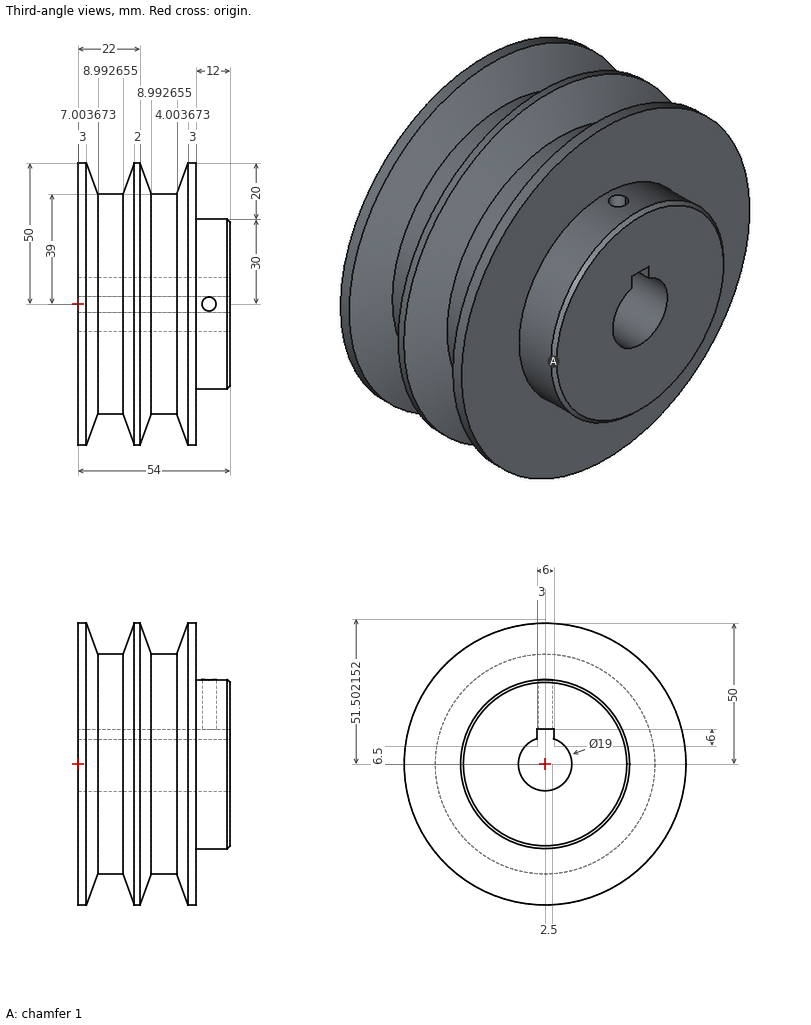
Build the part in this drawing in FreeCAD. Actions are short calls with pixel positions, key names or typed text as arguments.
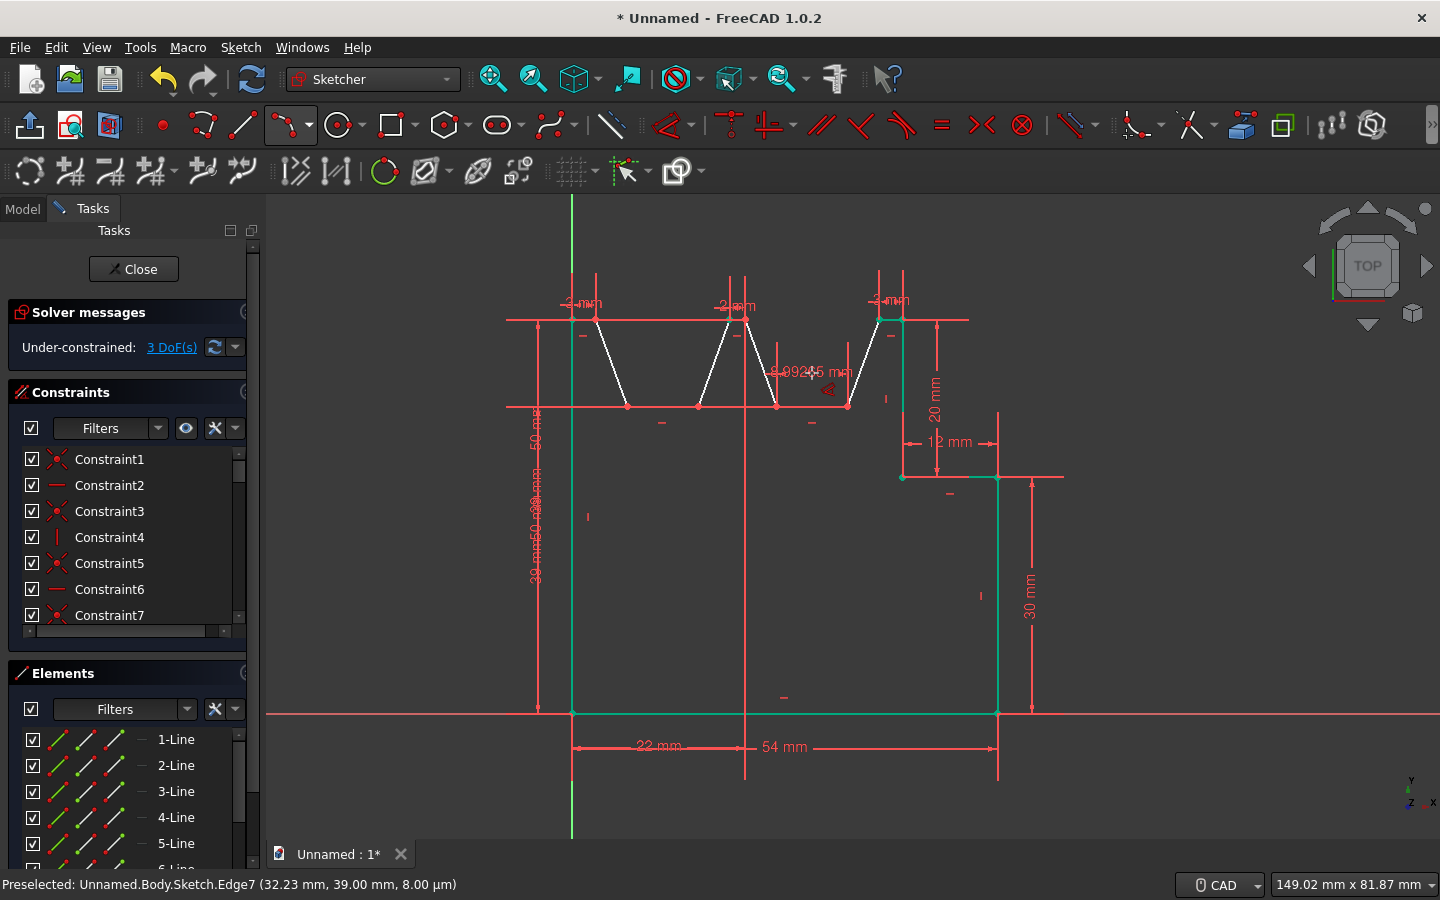
click(677, 407)
click(663, 373)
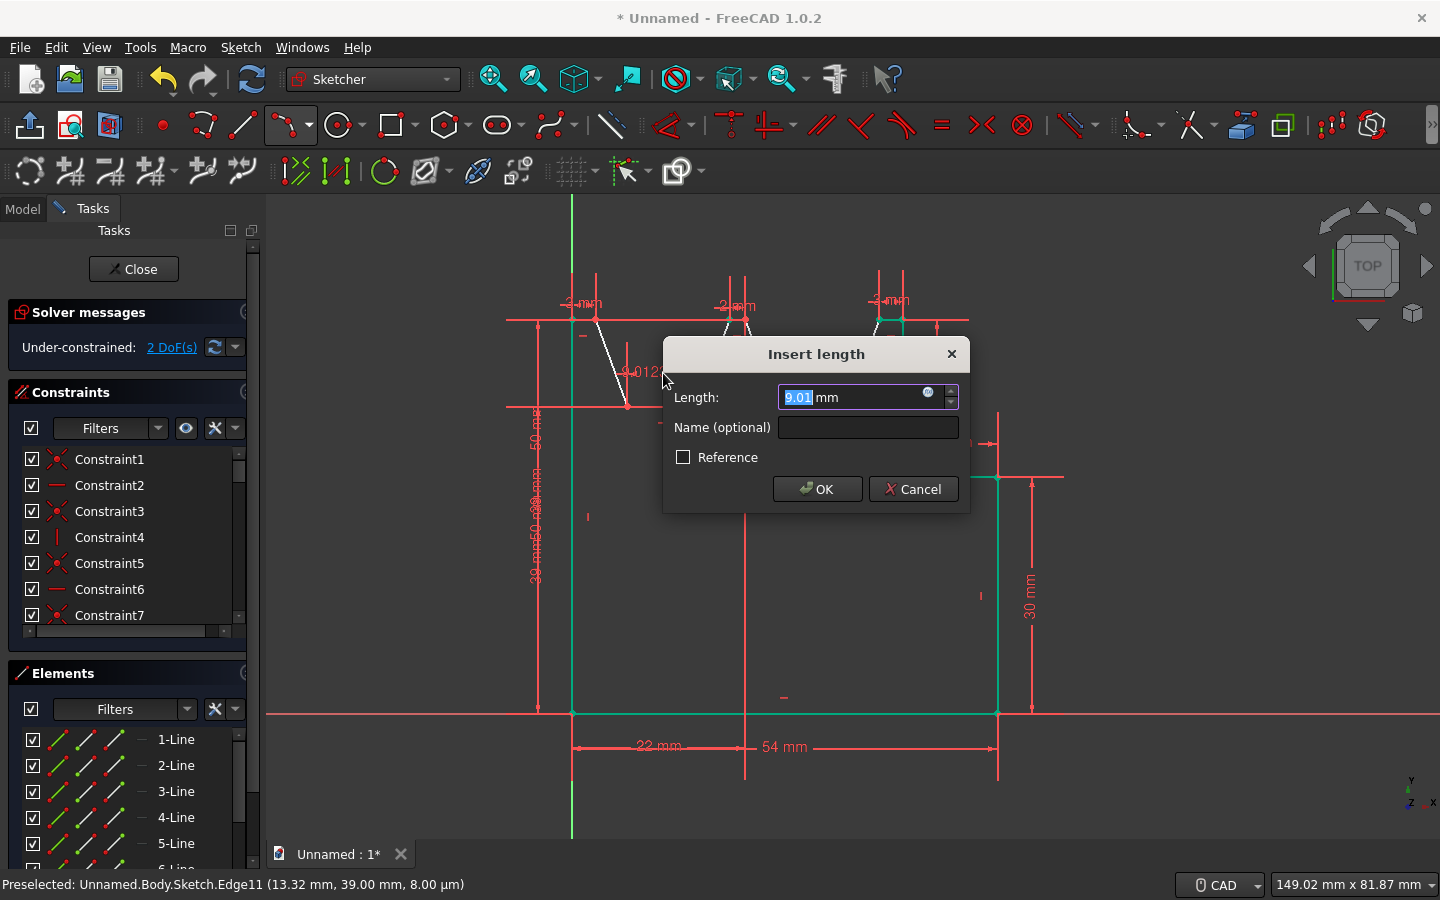
text(8.992655)
key(Return)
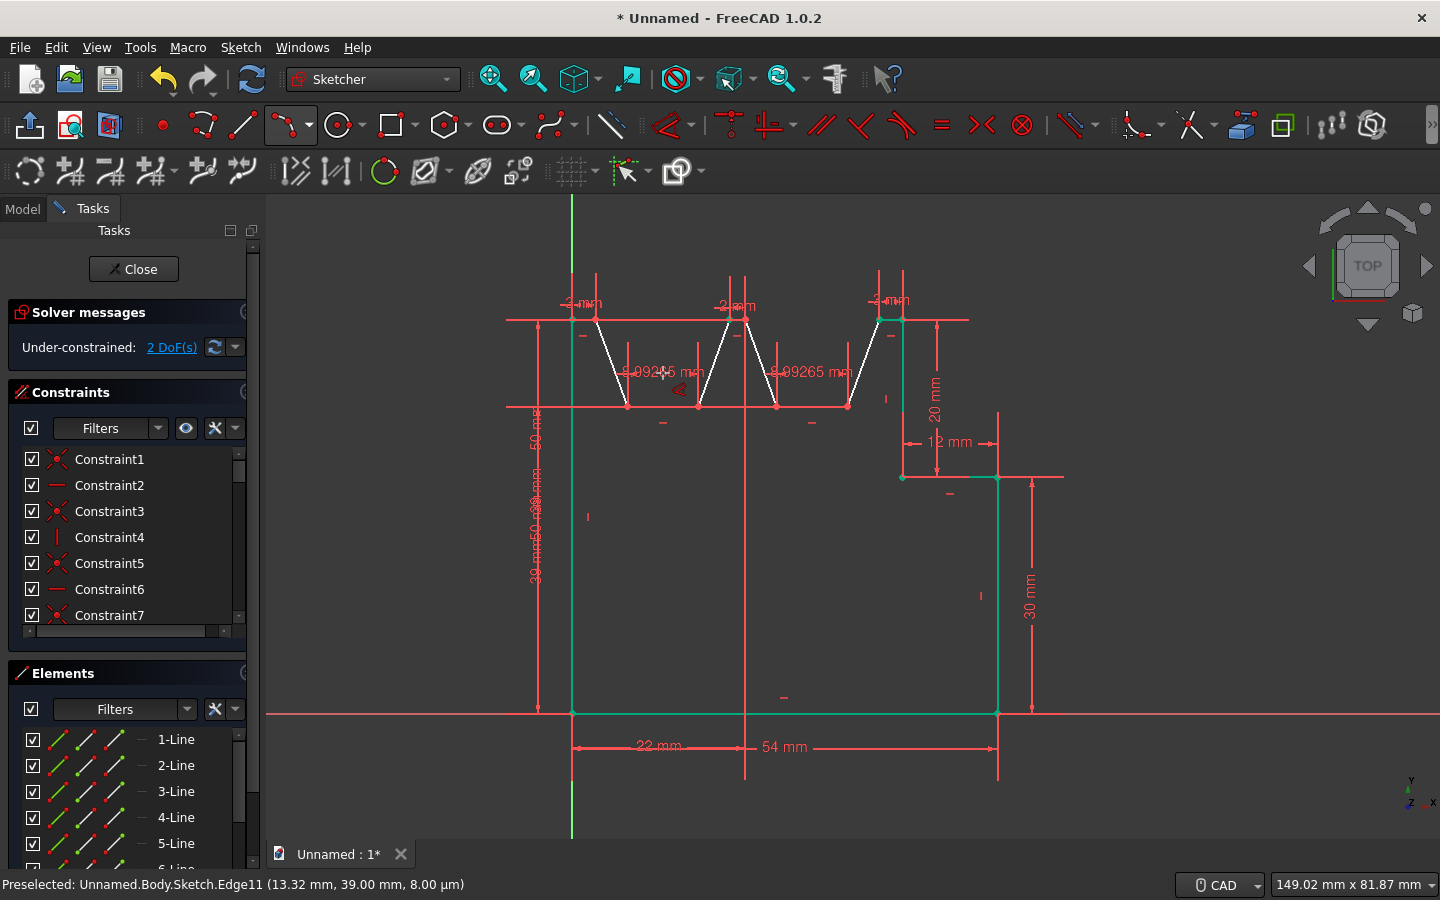
click(628, 407)
click(587, 748)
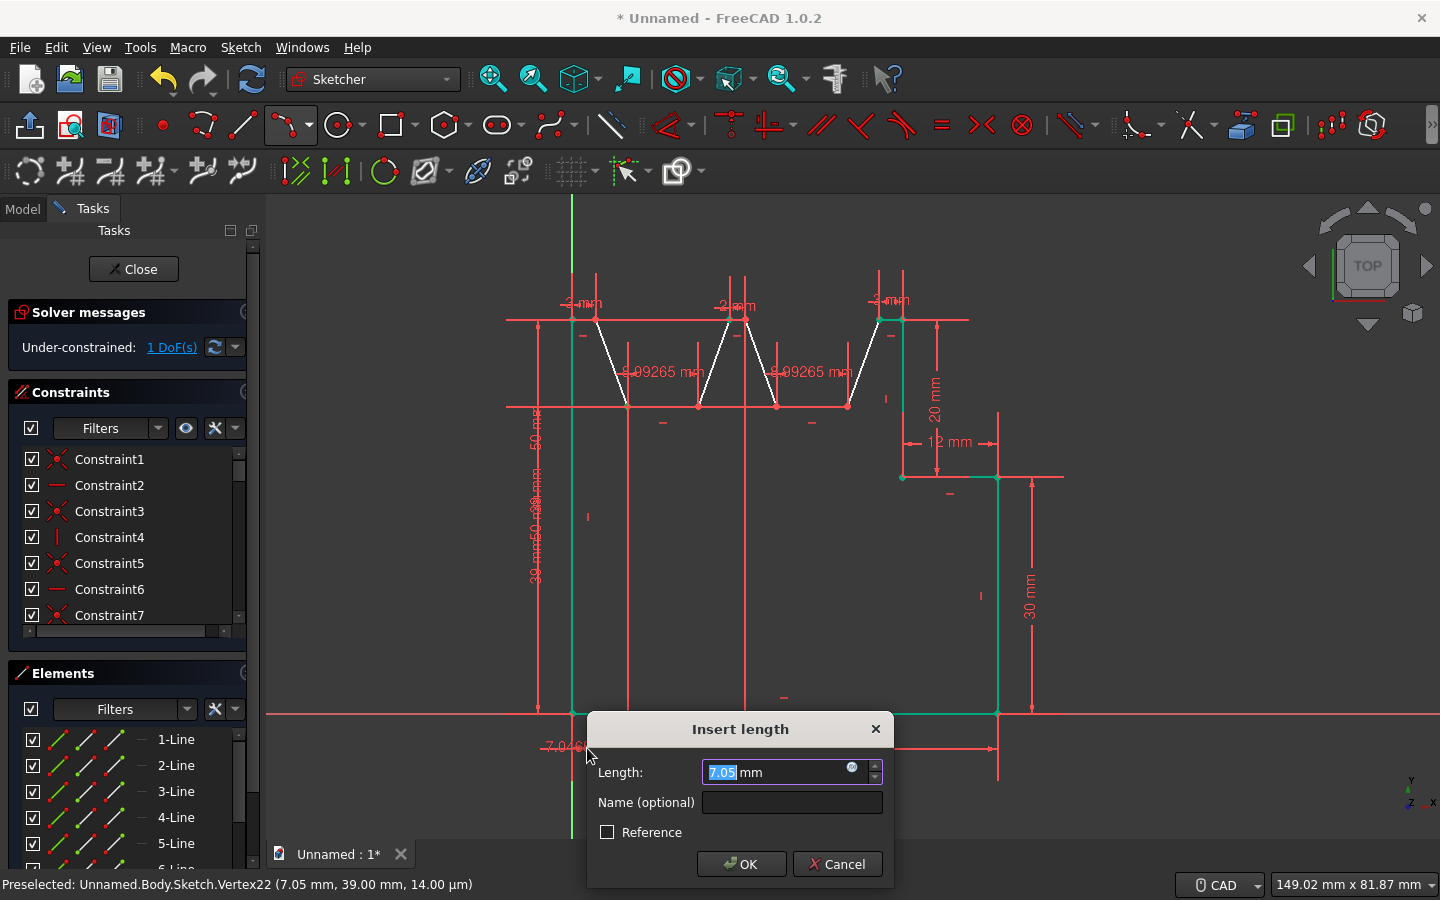
text(7.003673)
key(Return)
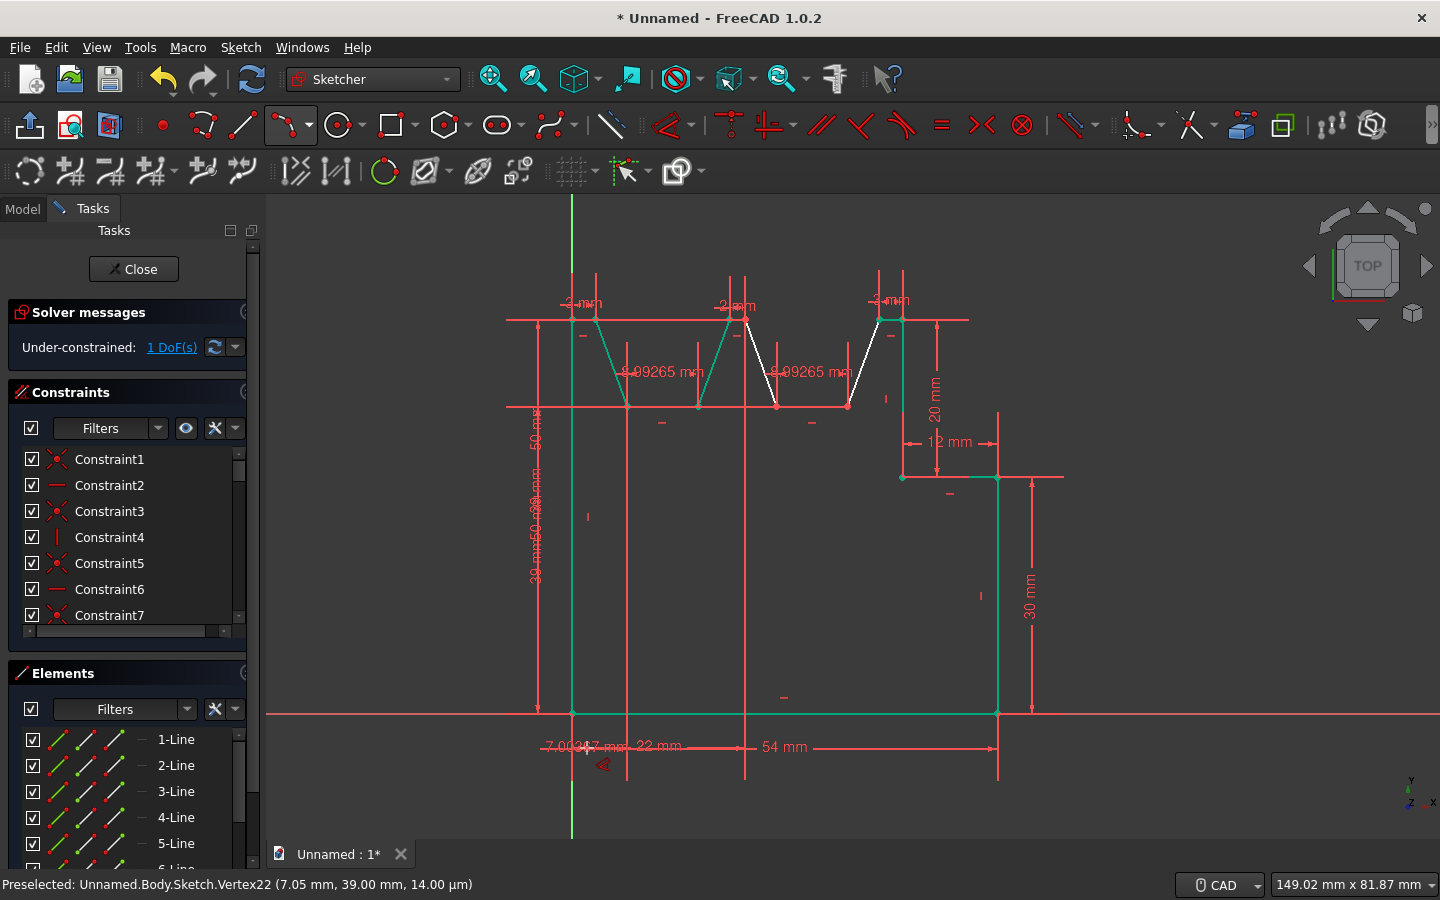
scroll(870, 346, up, 2)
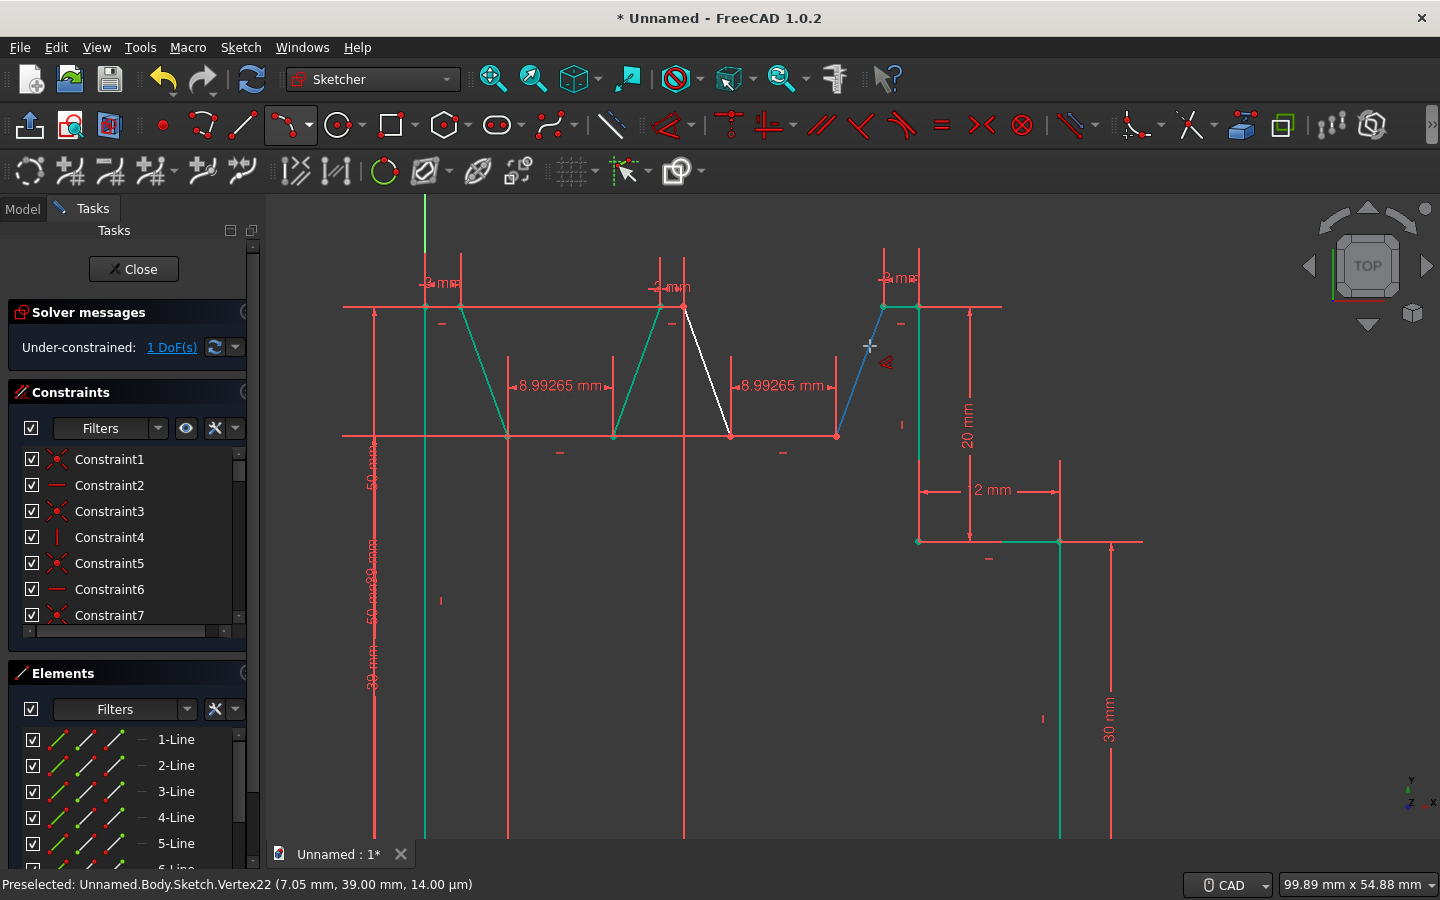
click(869, 346)
click(860, 470)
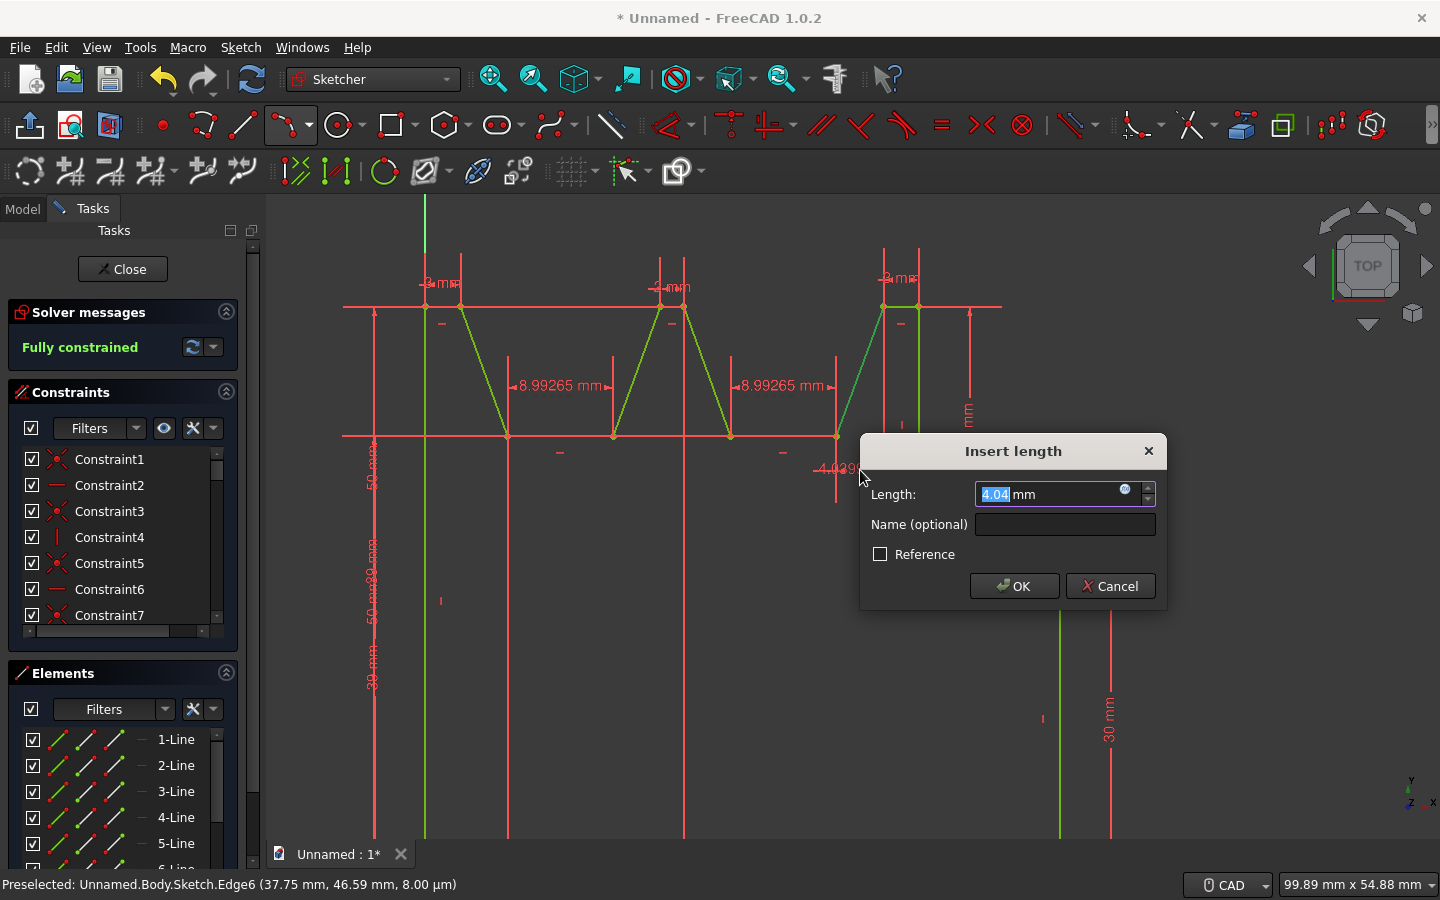
text(4.003673)
key(Return)
key(Escape)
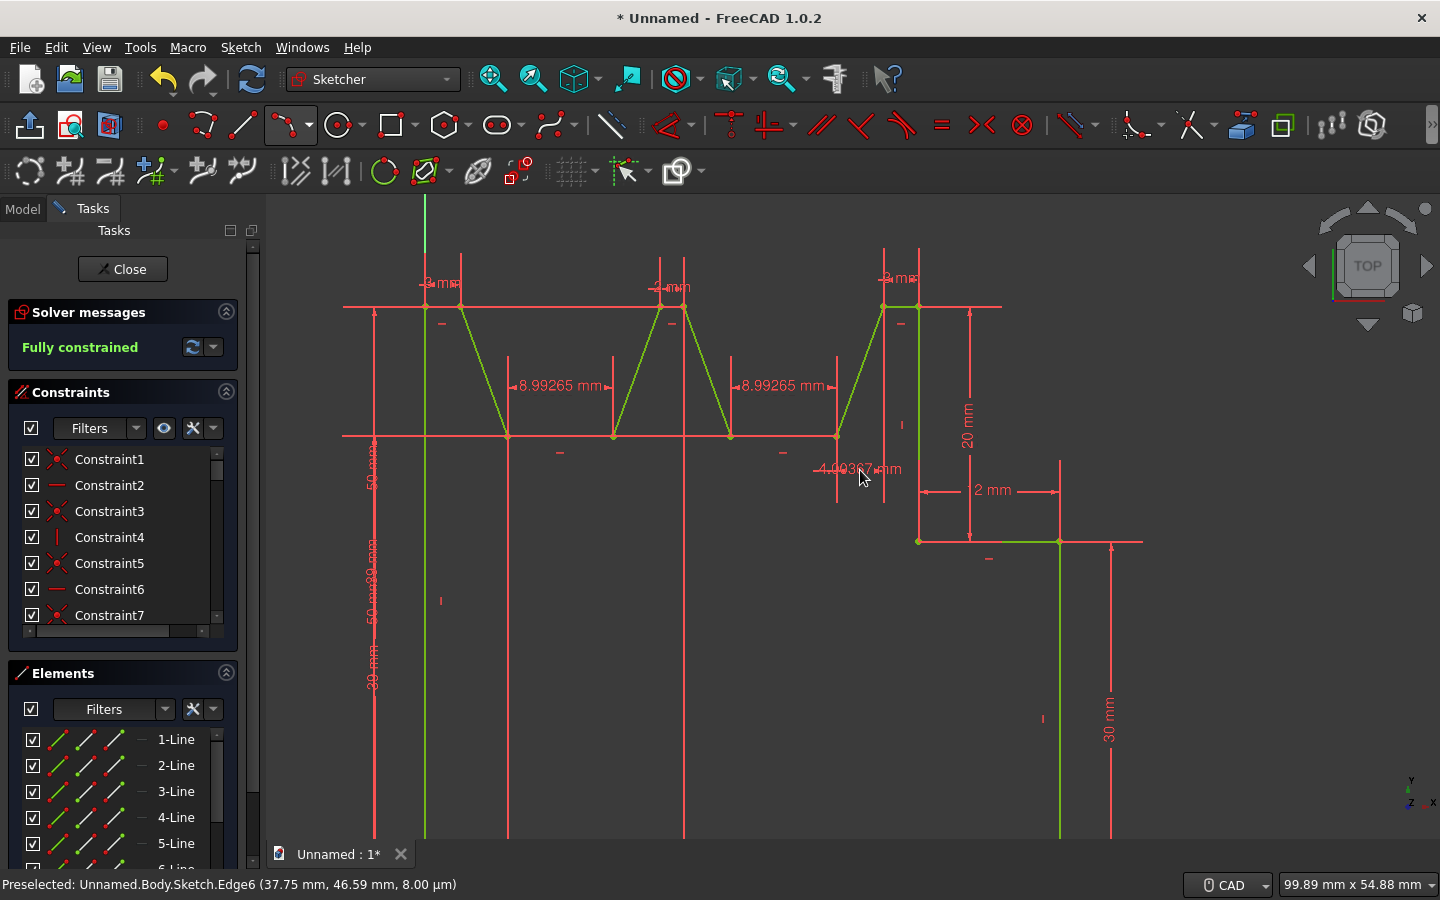
click(123, 269)